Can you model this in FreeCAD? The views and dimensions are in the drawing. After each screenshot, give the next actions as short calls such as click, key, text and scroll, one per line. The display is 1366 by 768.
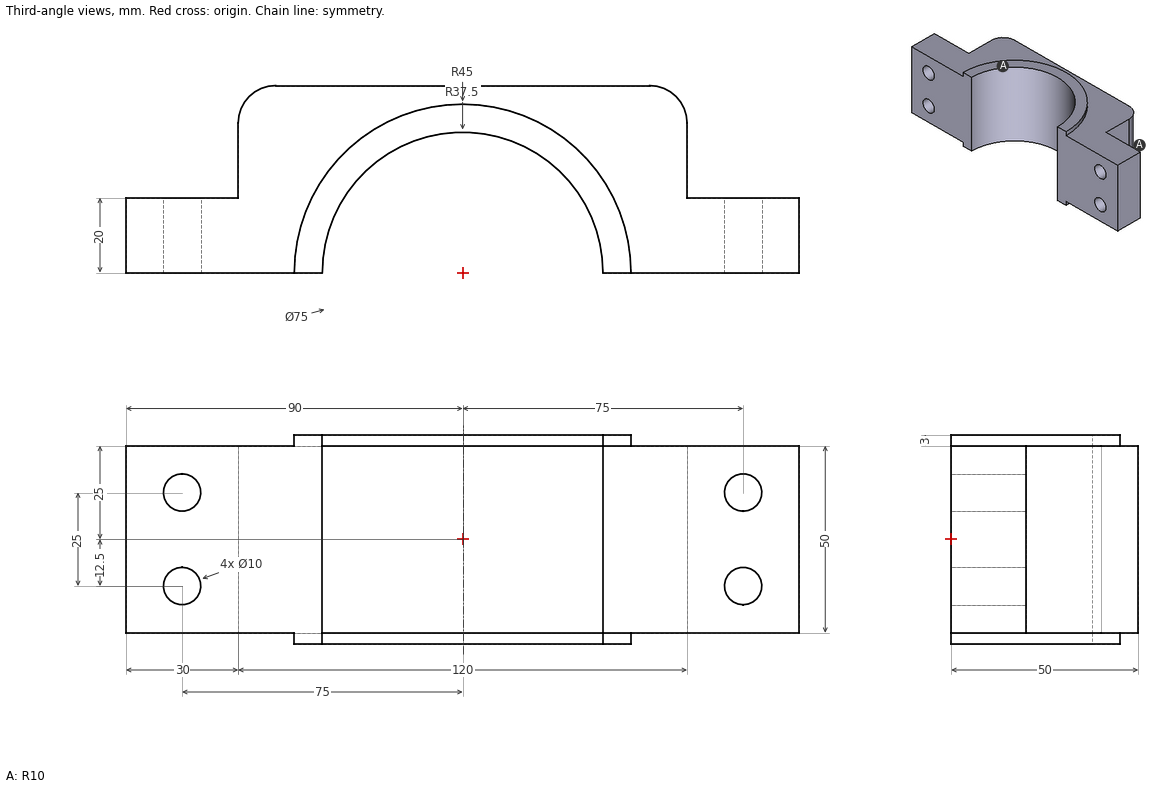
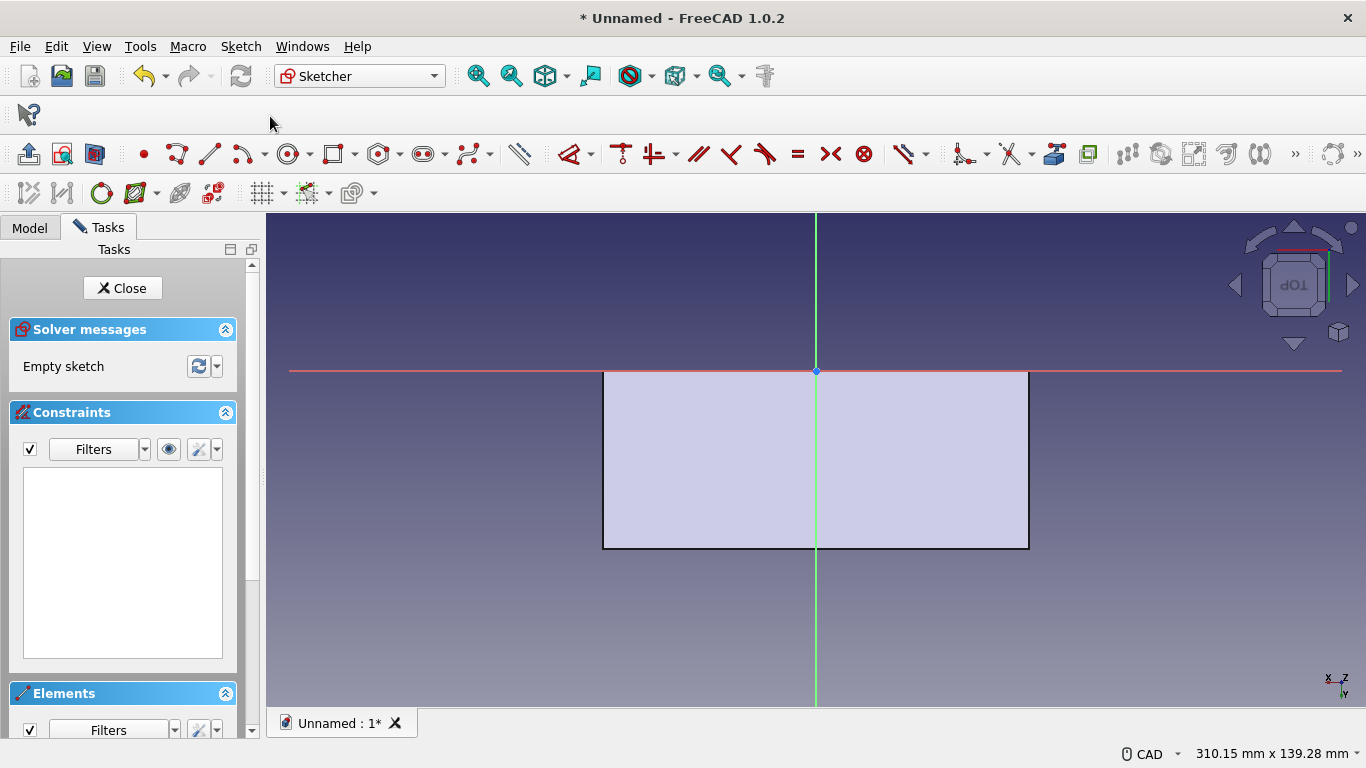
scroll(438, 679, down, 1)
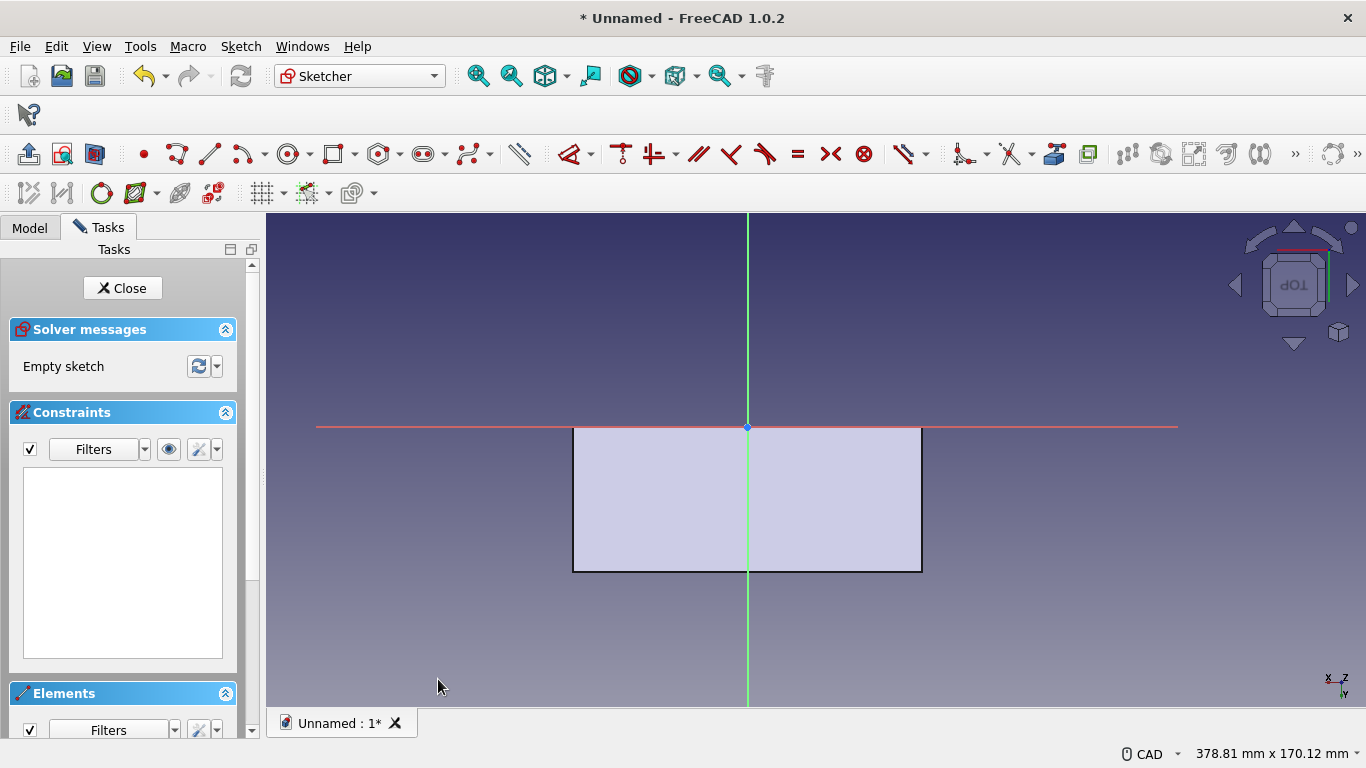
scroll(748, 361, up, 2)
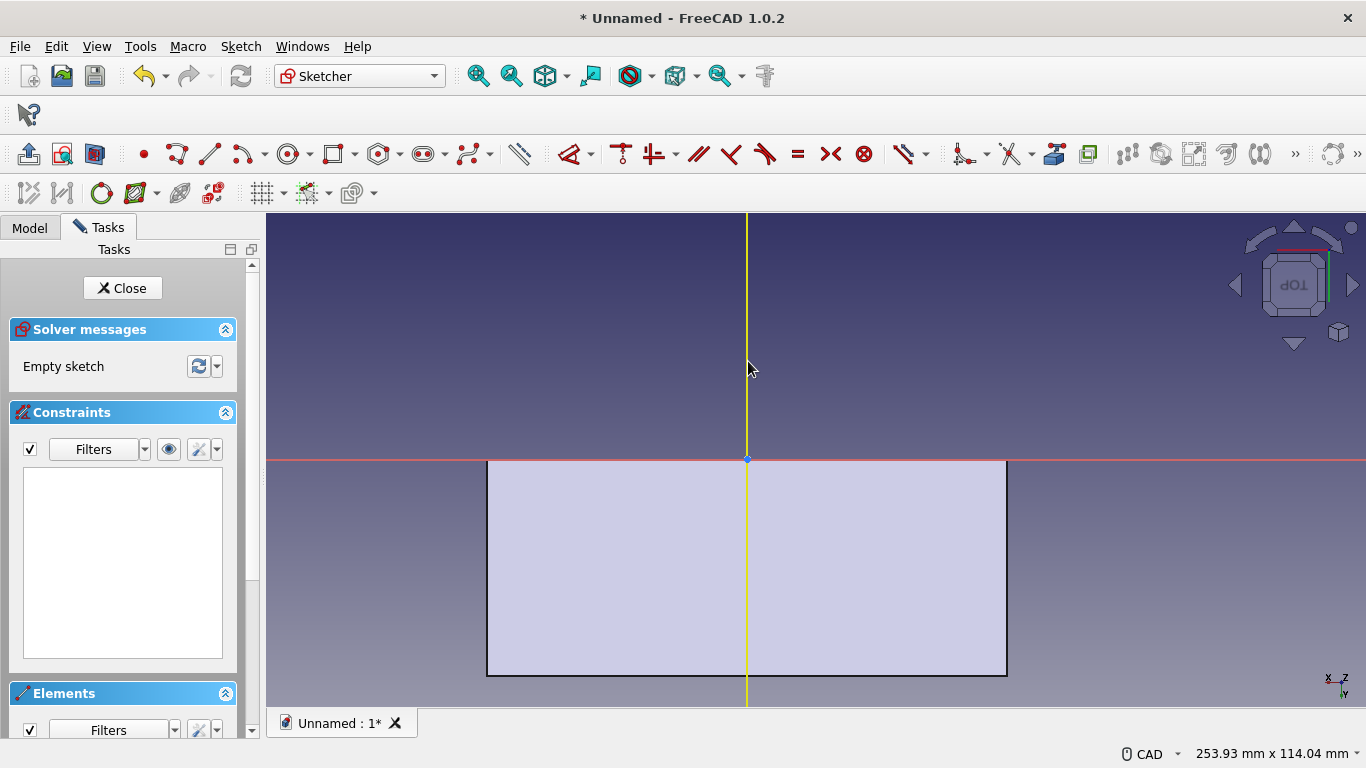
click(288, 154)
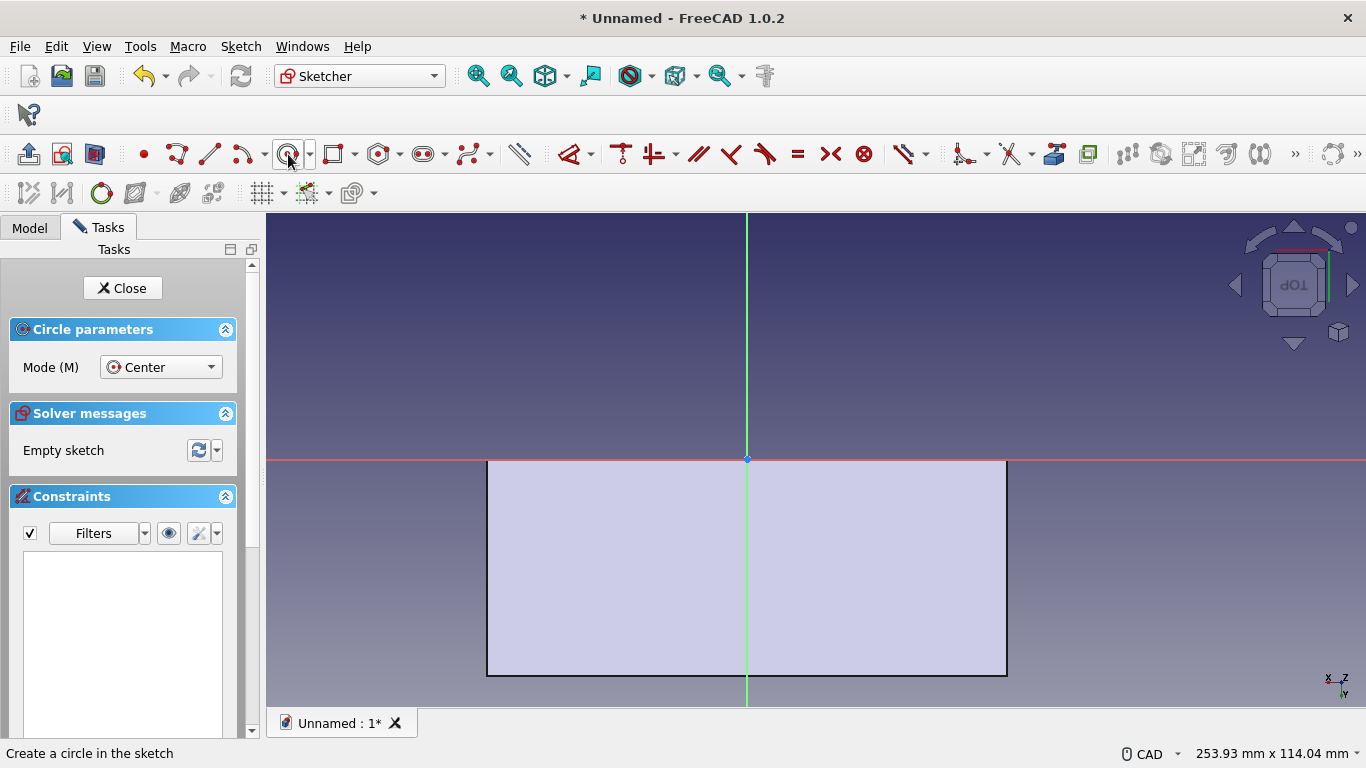
click(747, 460)
click(862, 345)
key(Escape)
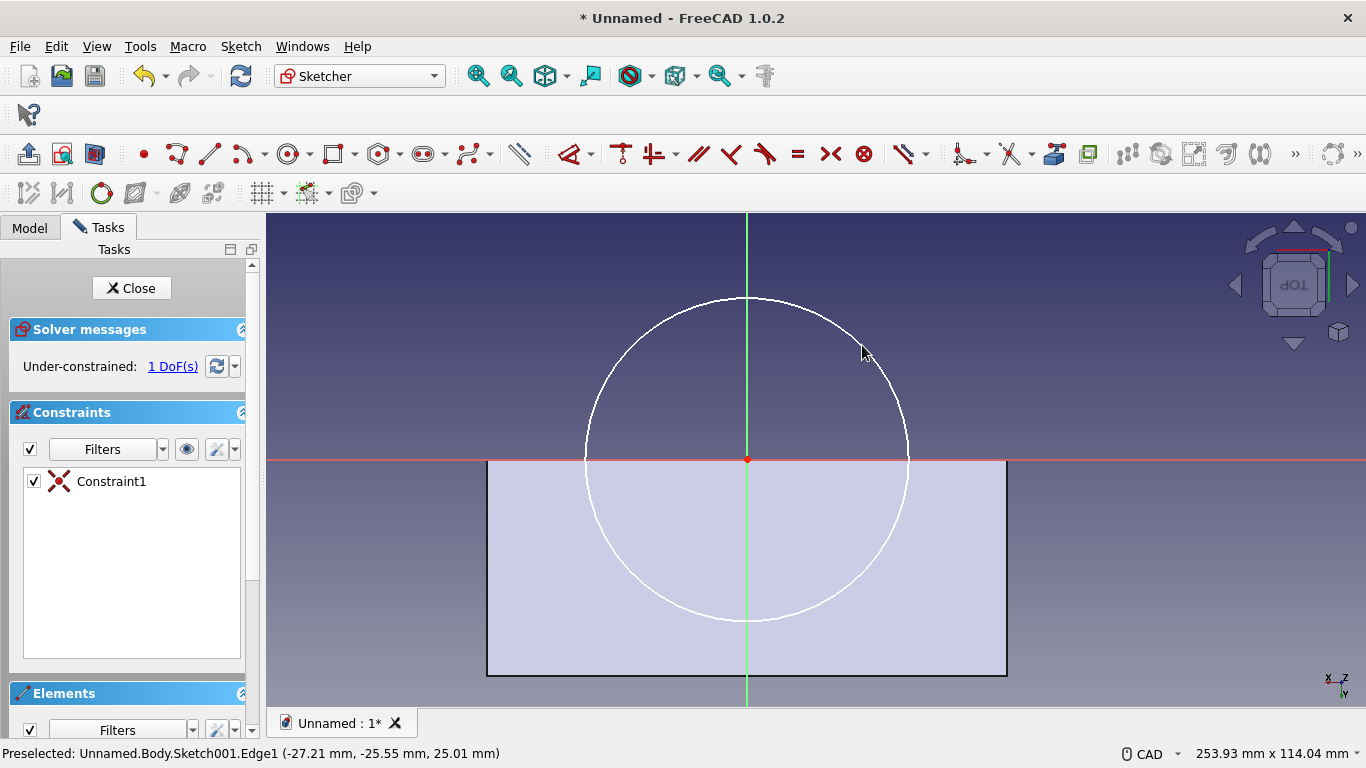
click(861, 345)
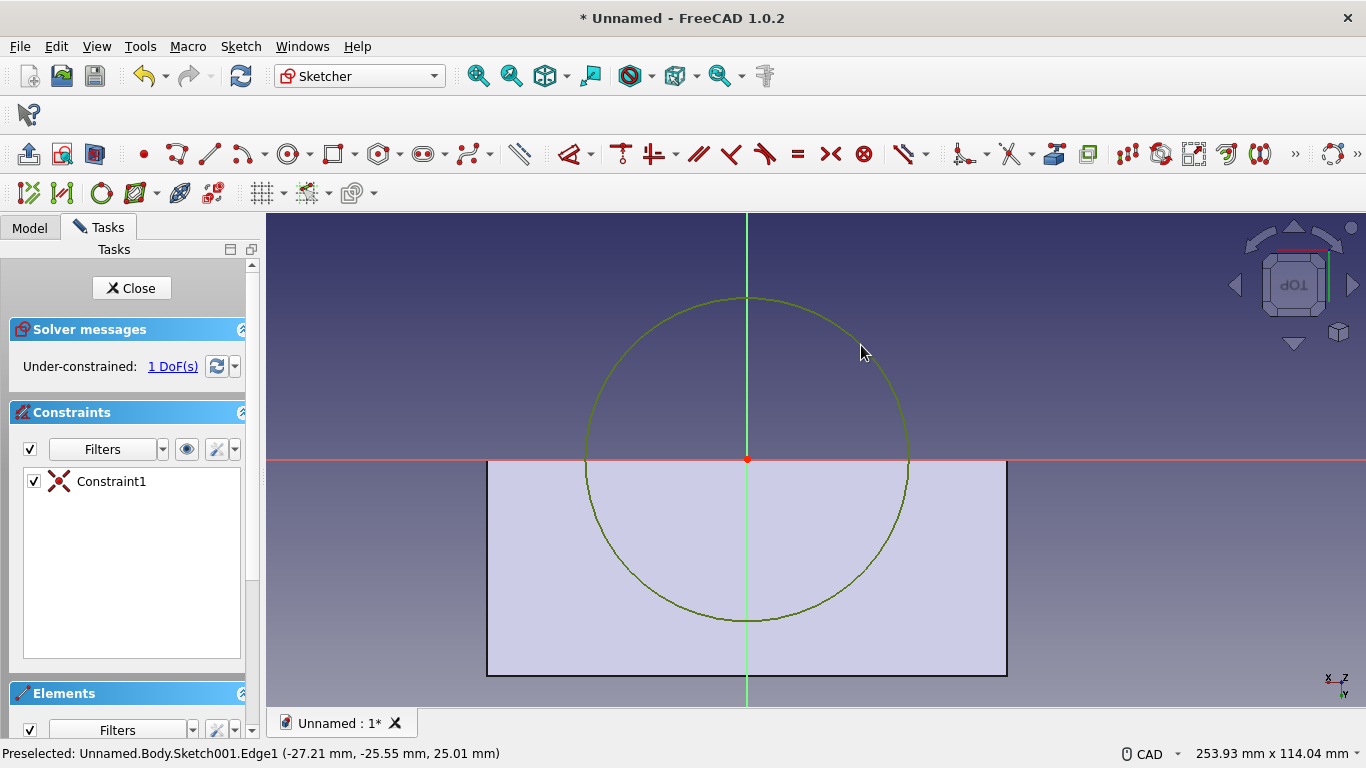
key(k)
key(o)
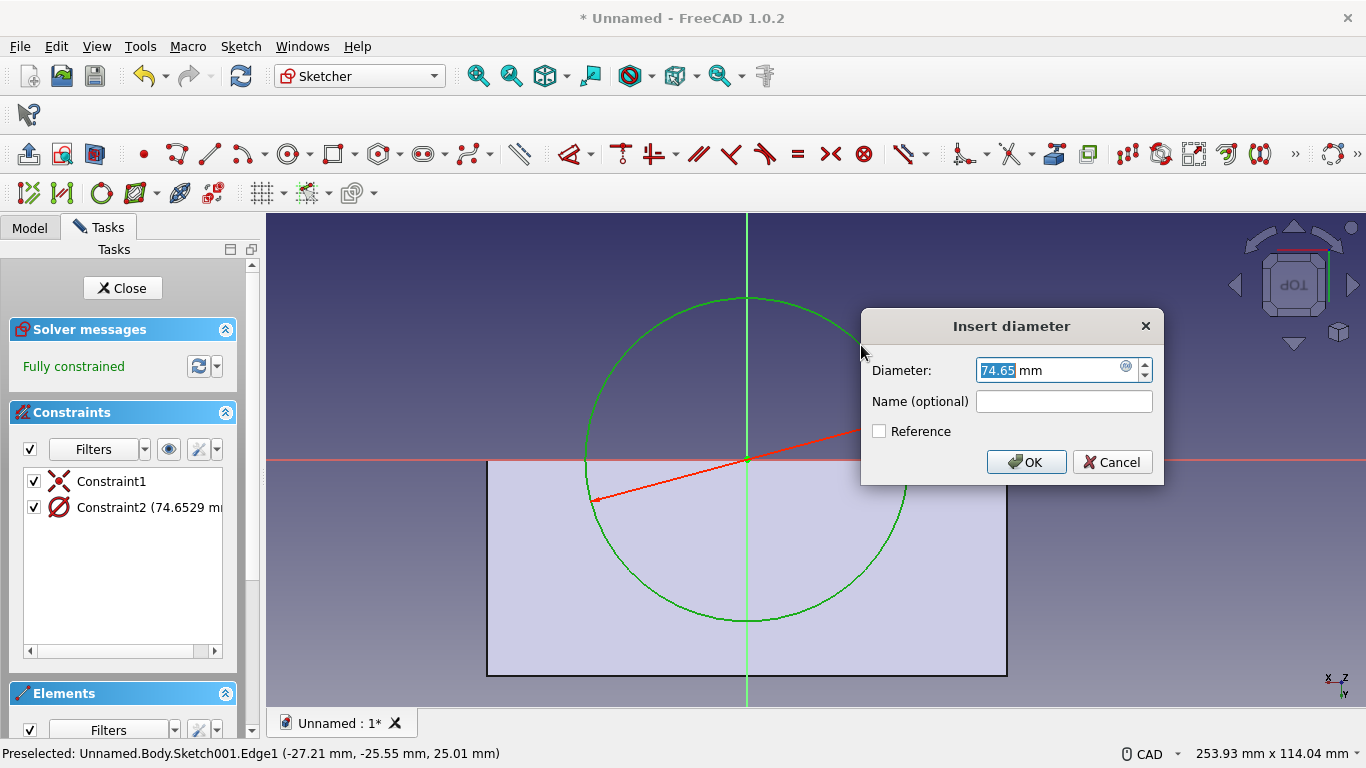
text(75)
key(Return)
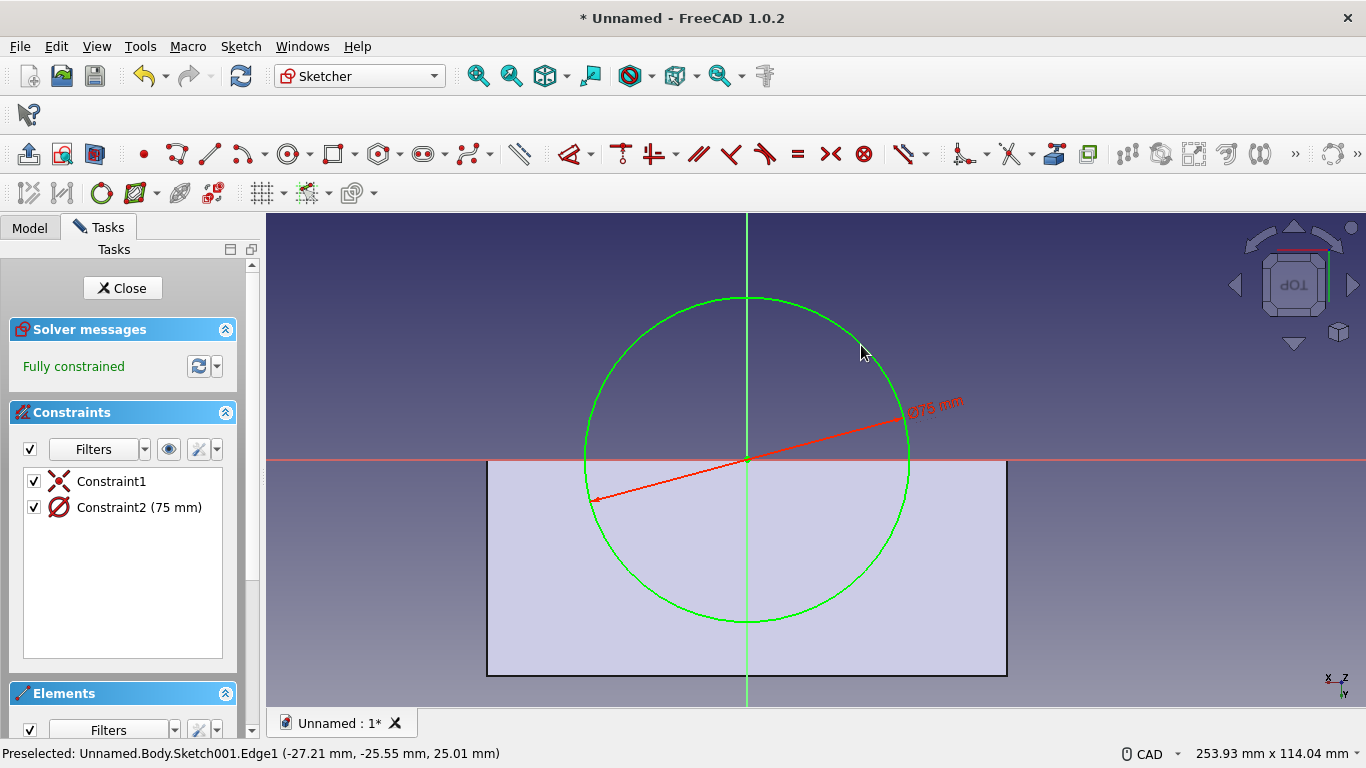
click(123, 288)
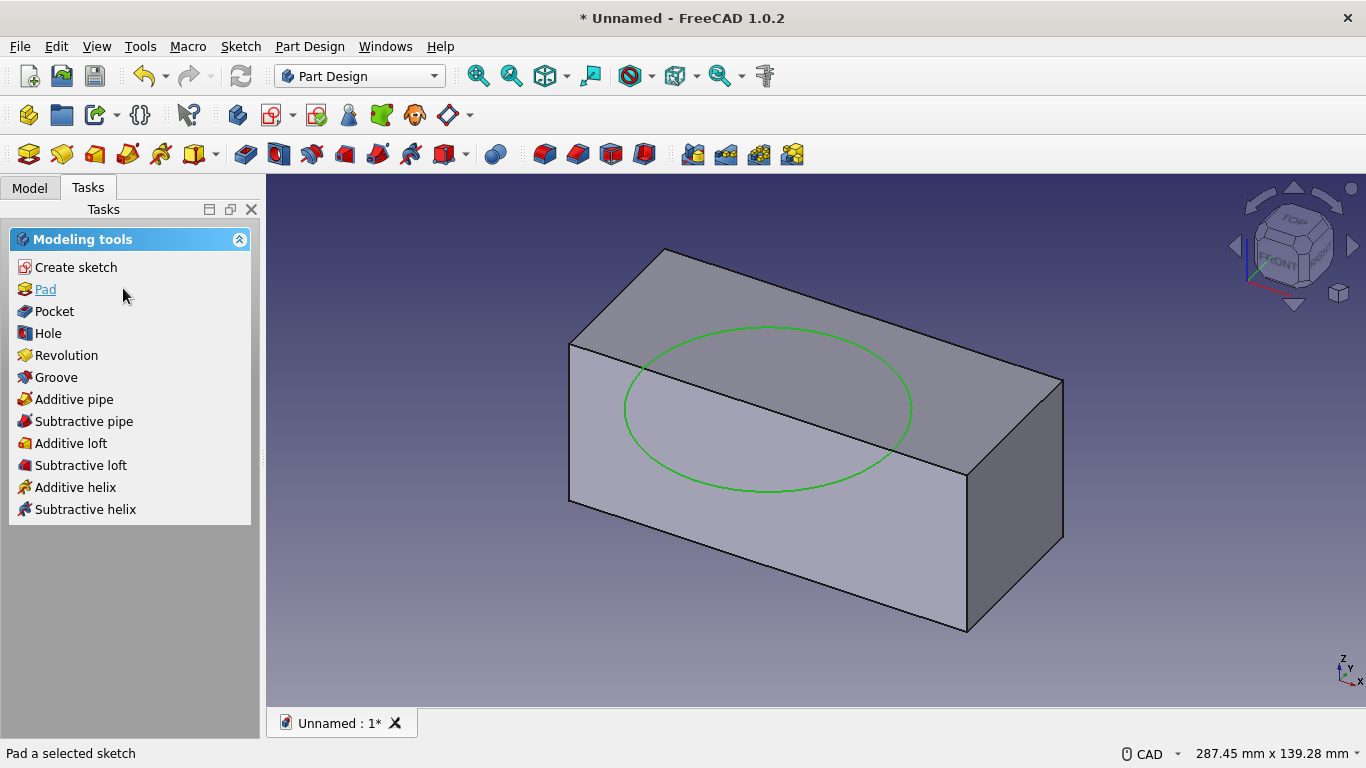
click(246, 154)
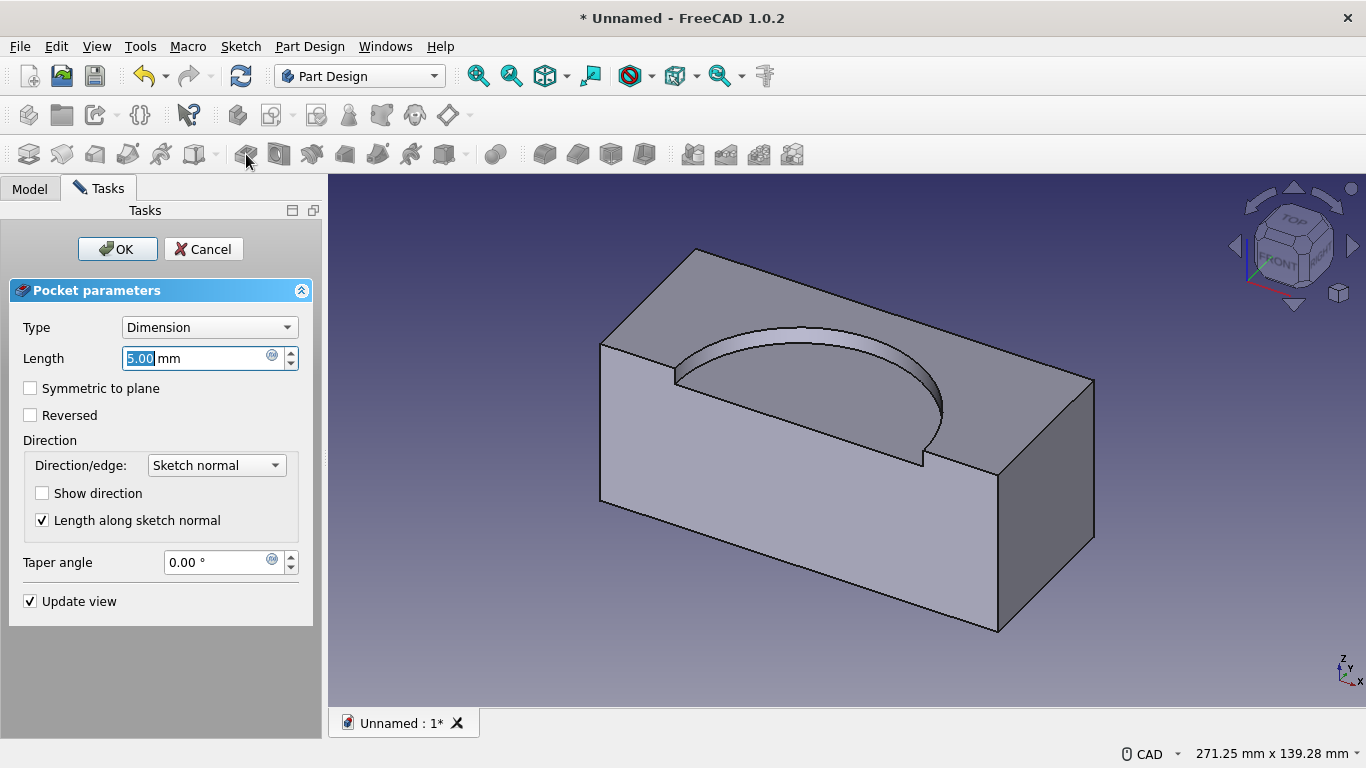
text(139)
key(Tab)